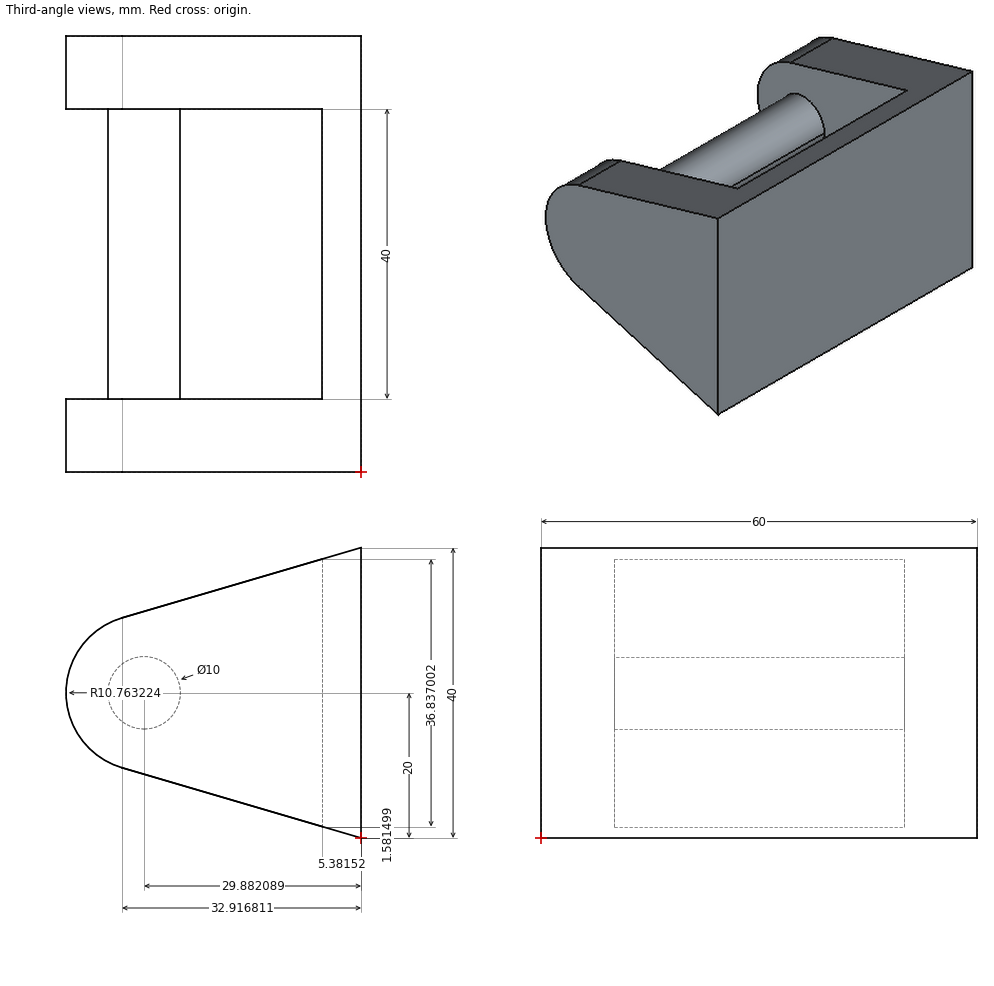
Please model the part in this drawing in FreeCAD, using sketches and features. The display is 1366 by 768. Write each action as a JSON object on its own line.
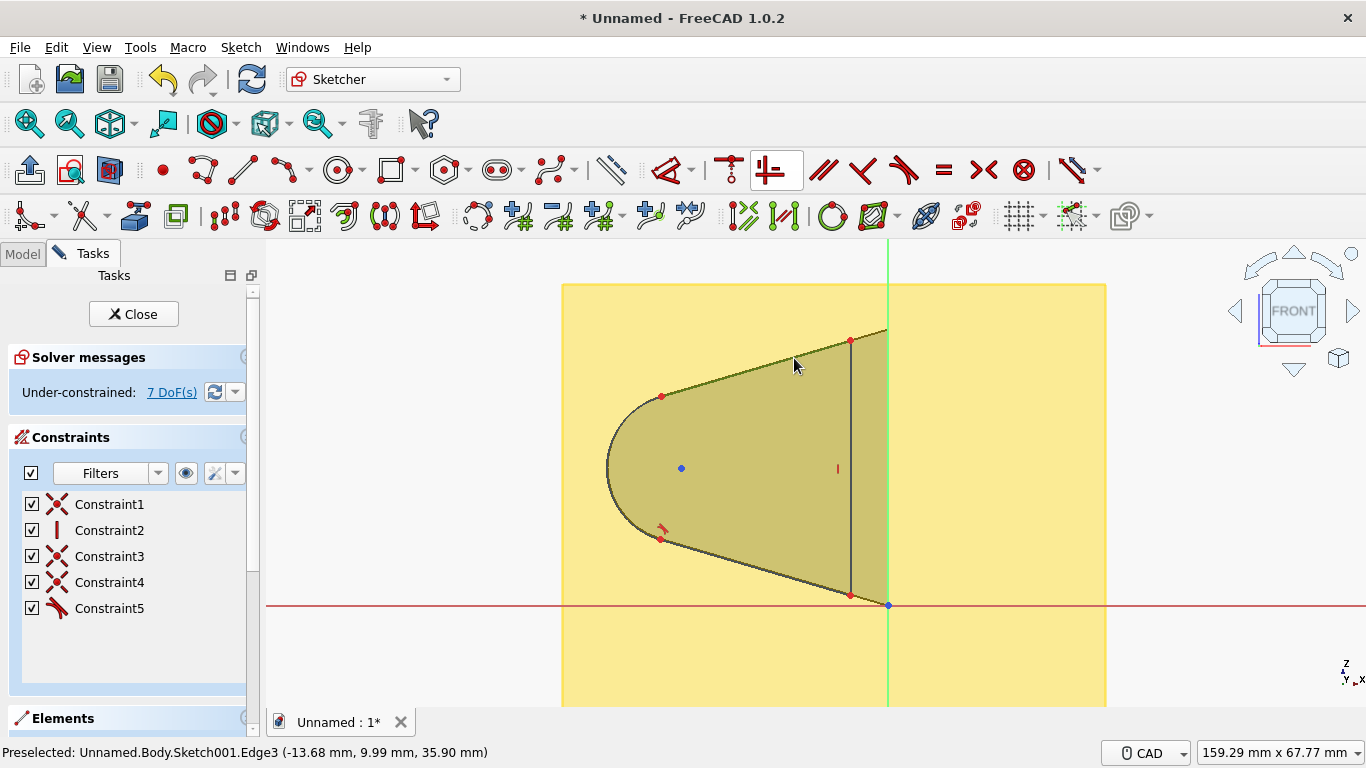
{"action": "left_click", "coordinate": [617, 431]}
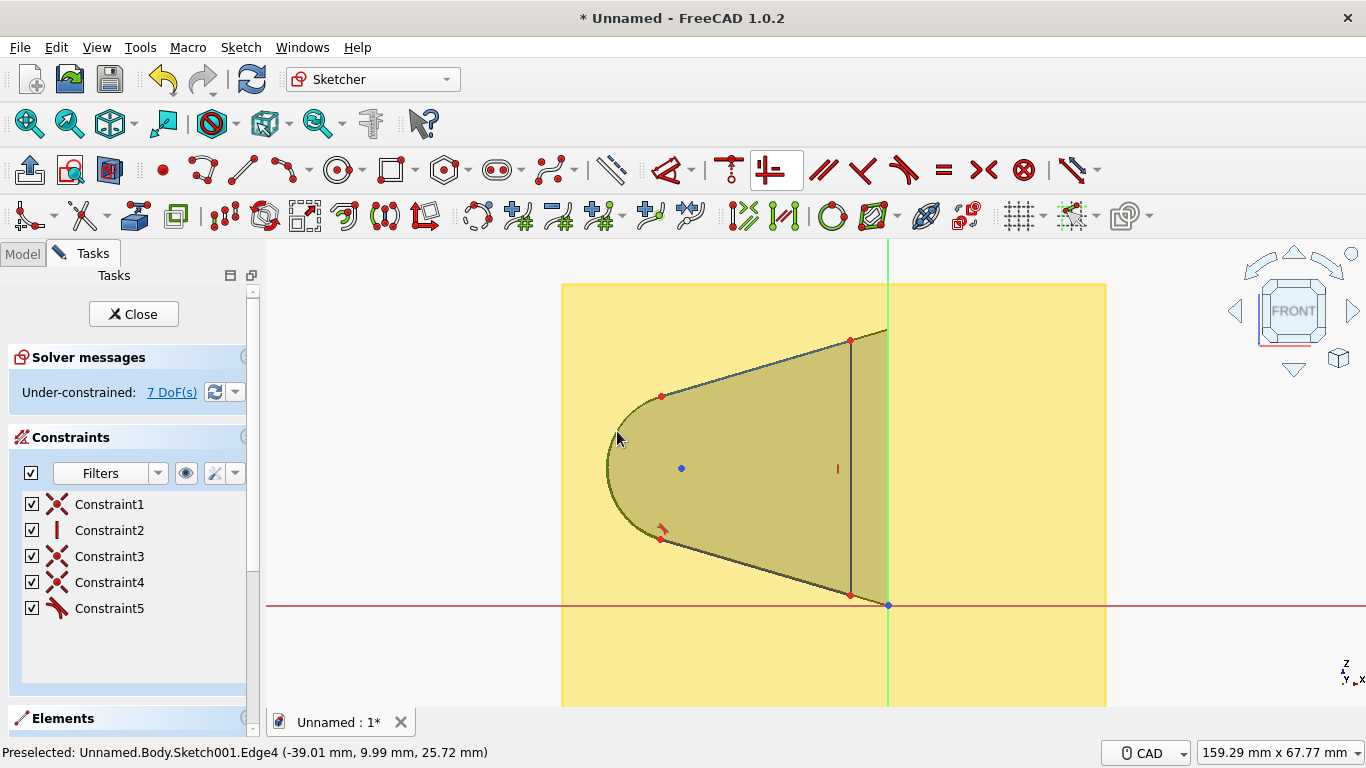
{"action": "left_click", "coordinate": [904, 170]}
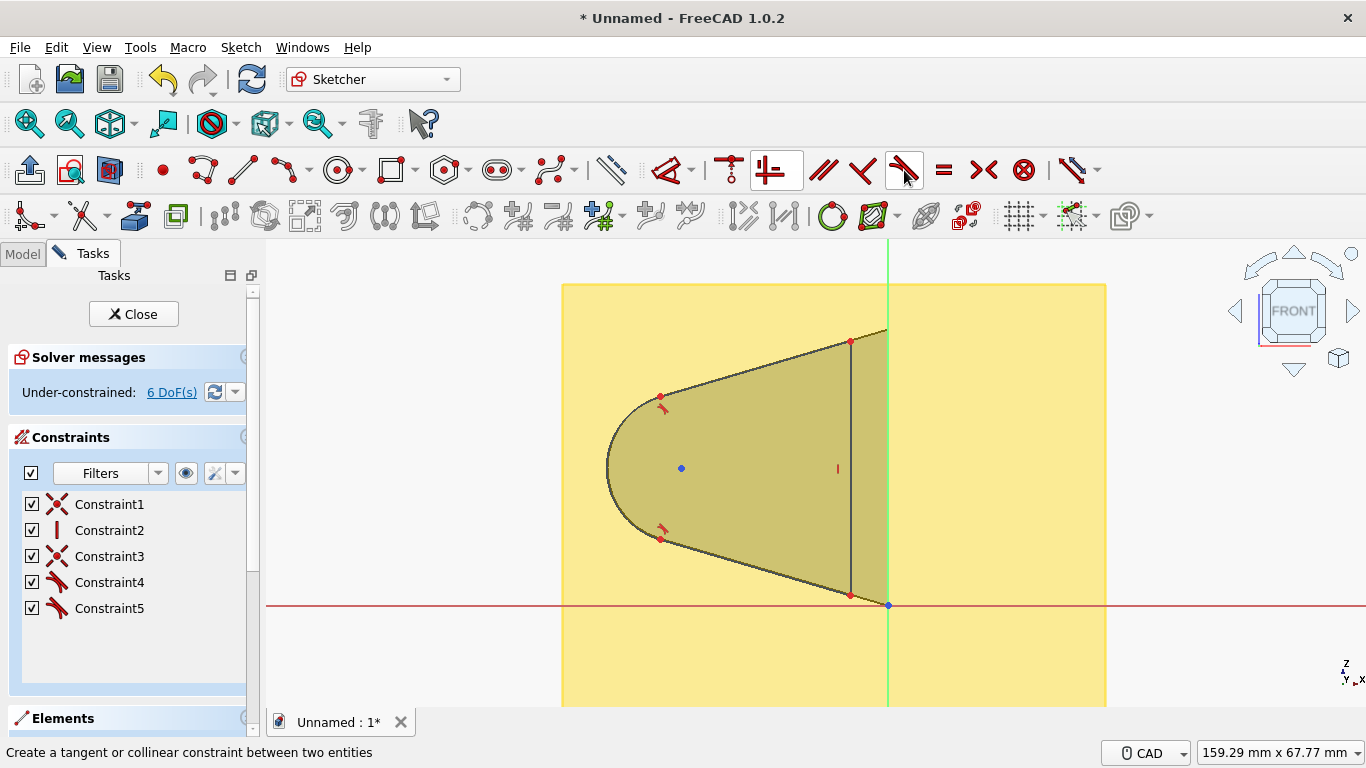
{"action": "left_click", "coordinate": [666, 170]}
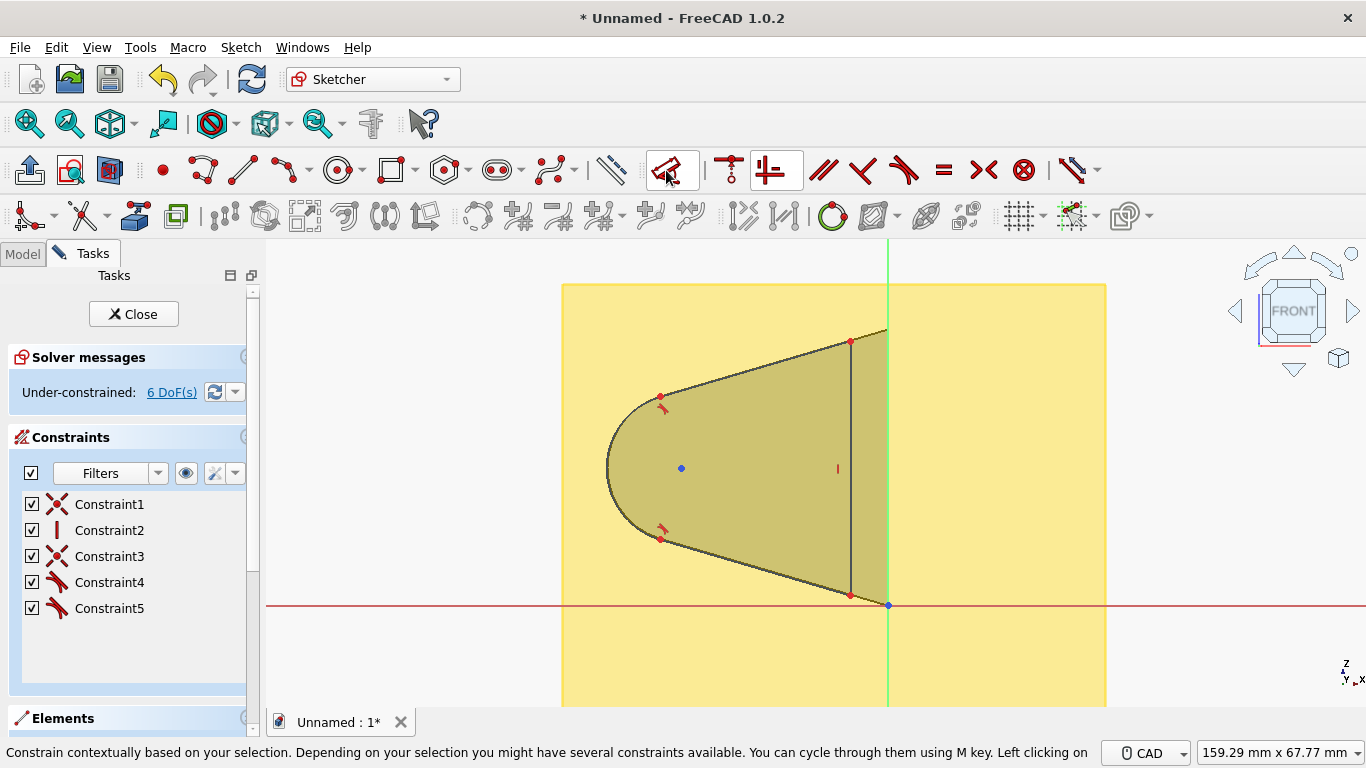
{"action": "left_click", "coordinate": [616, 432]}
{"action": "left_click", "coordinate": [588, 416]}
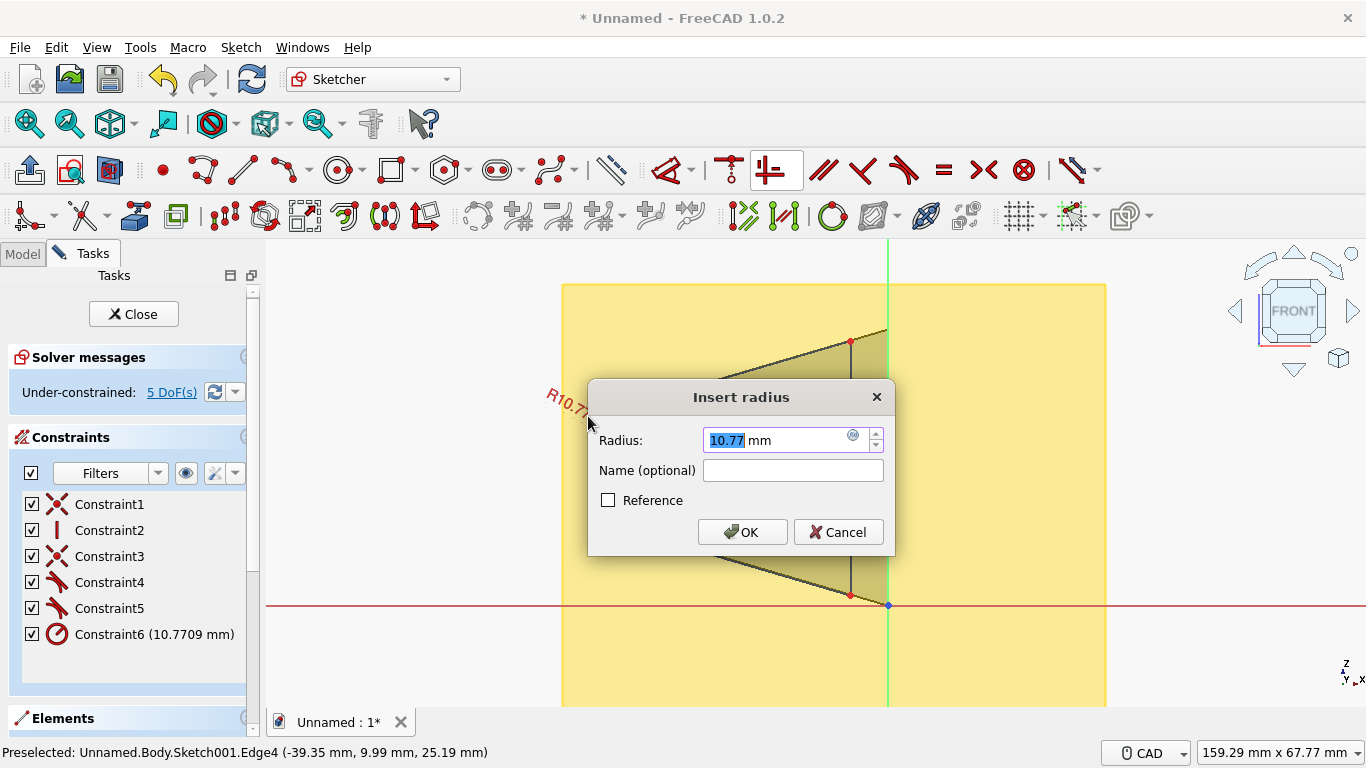
{"action": "type", "text": "10.763224"}
{"action": "key", "text": "Return"}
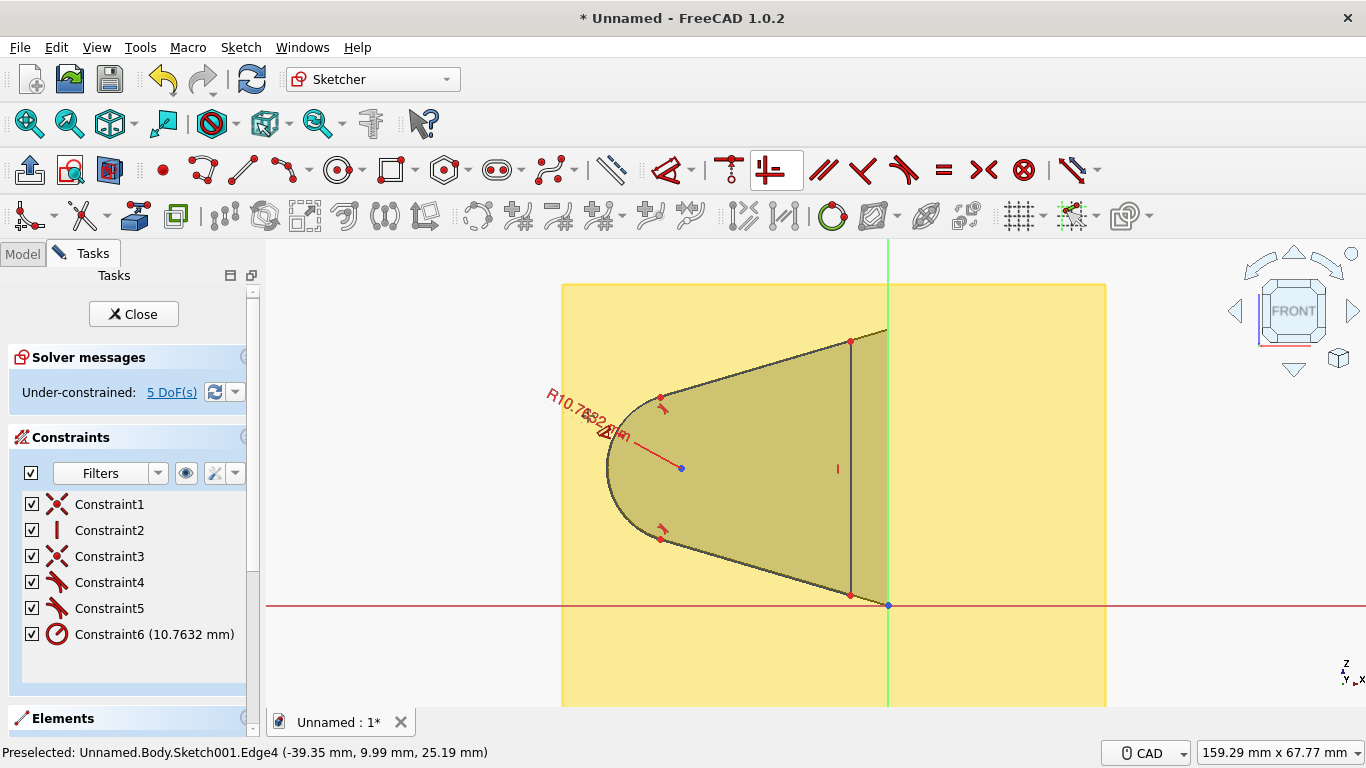
{"action": "left_click", "coordinate": [681, 468]}
{"action": "left_click", "coordinate": [922, 537]}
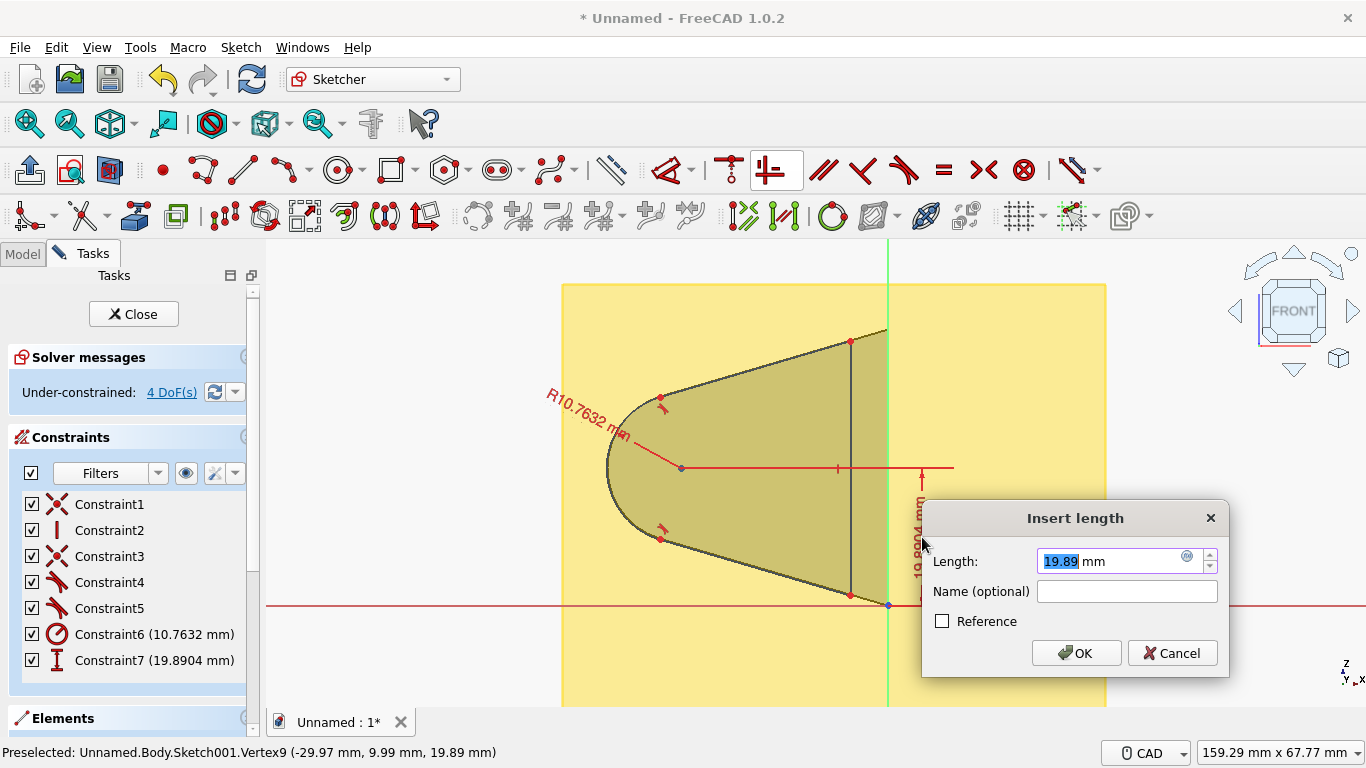
{"action": "type", "text": "20"}
{"action": "key", "text": "Return"}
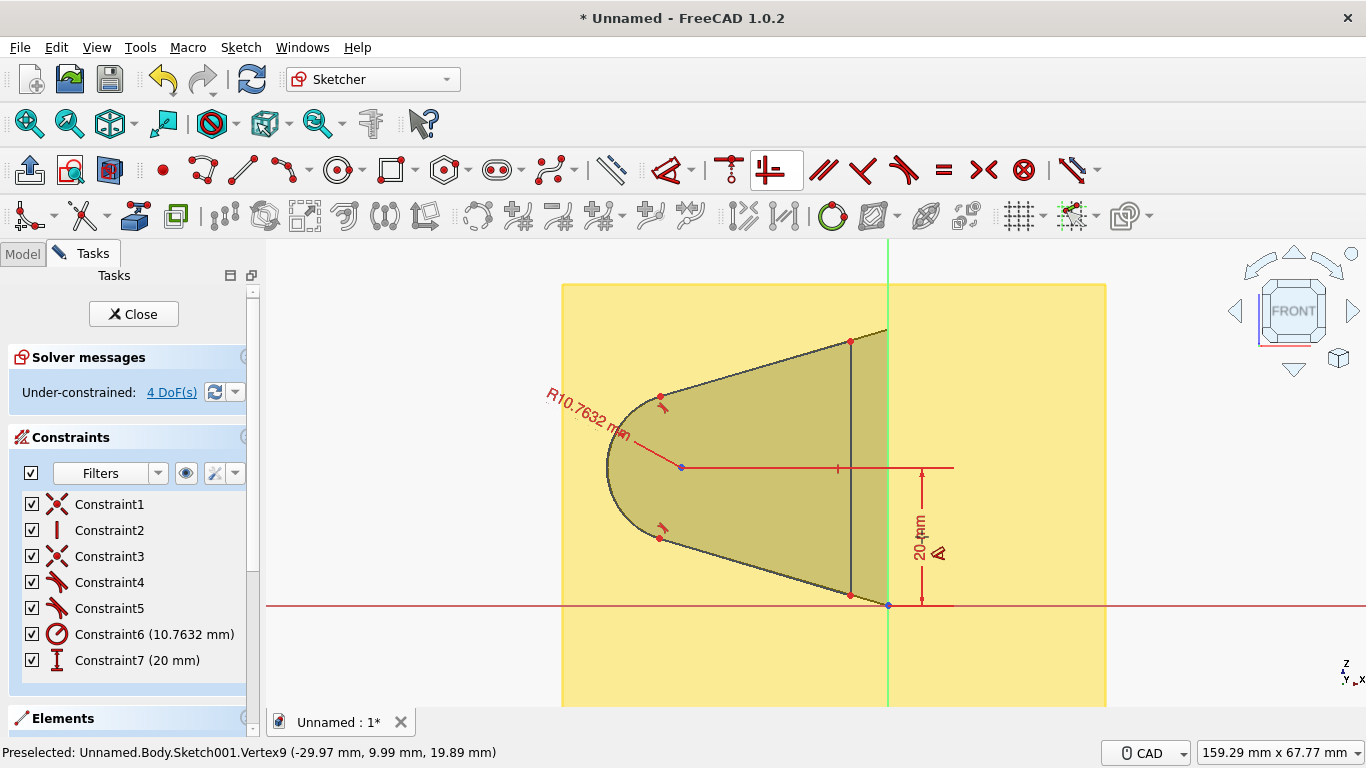
{"action": "left_click", "coordinate": [851, 596]}
{"action": "left_click", "coordinate": [869, 640]}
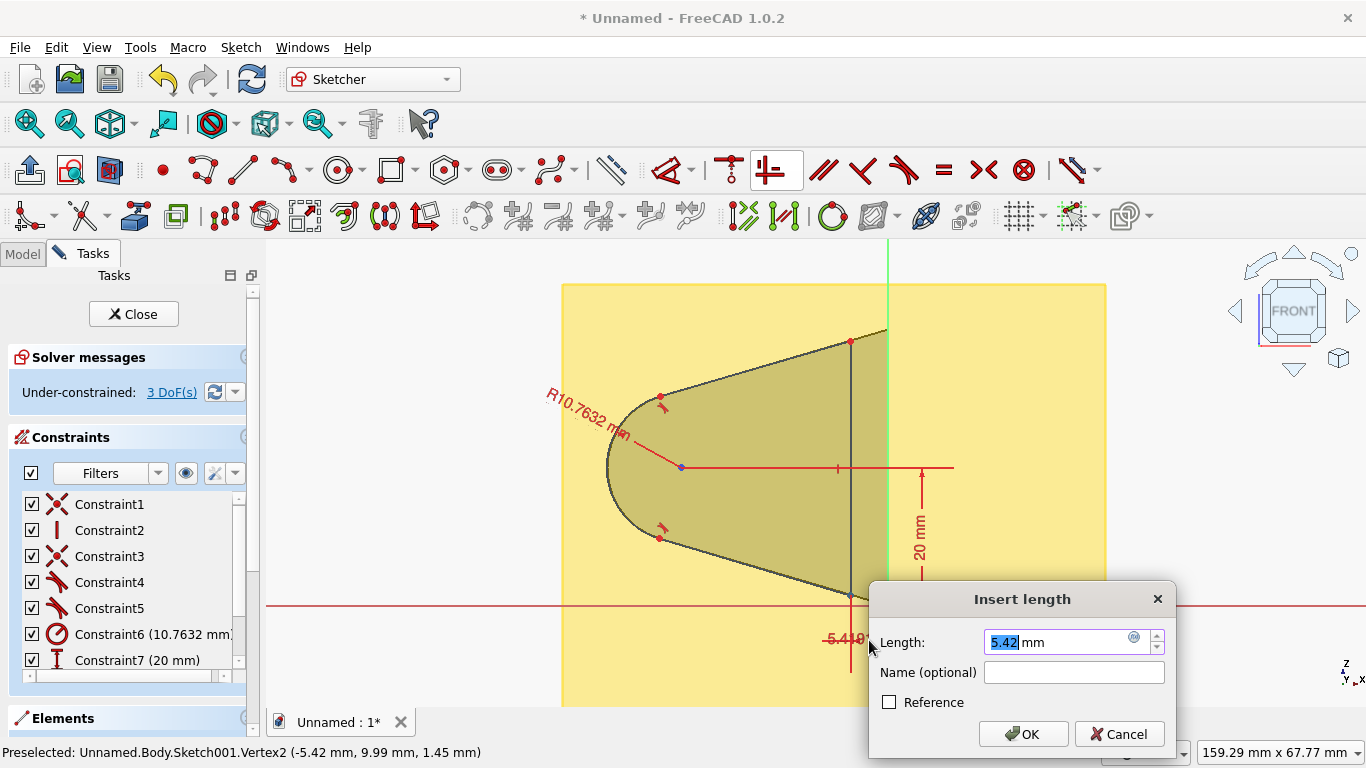
{"action": "type", "text": "5.38152"}
{"action": "key", "text": "Return"}